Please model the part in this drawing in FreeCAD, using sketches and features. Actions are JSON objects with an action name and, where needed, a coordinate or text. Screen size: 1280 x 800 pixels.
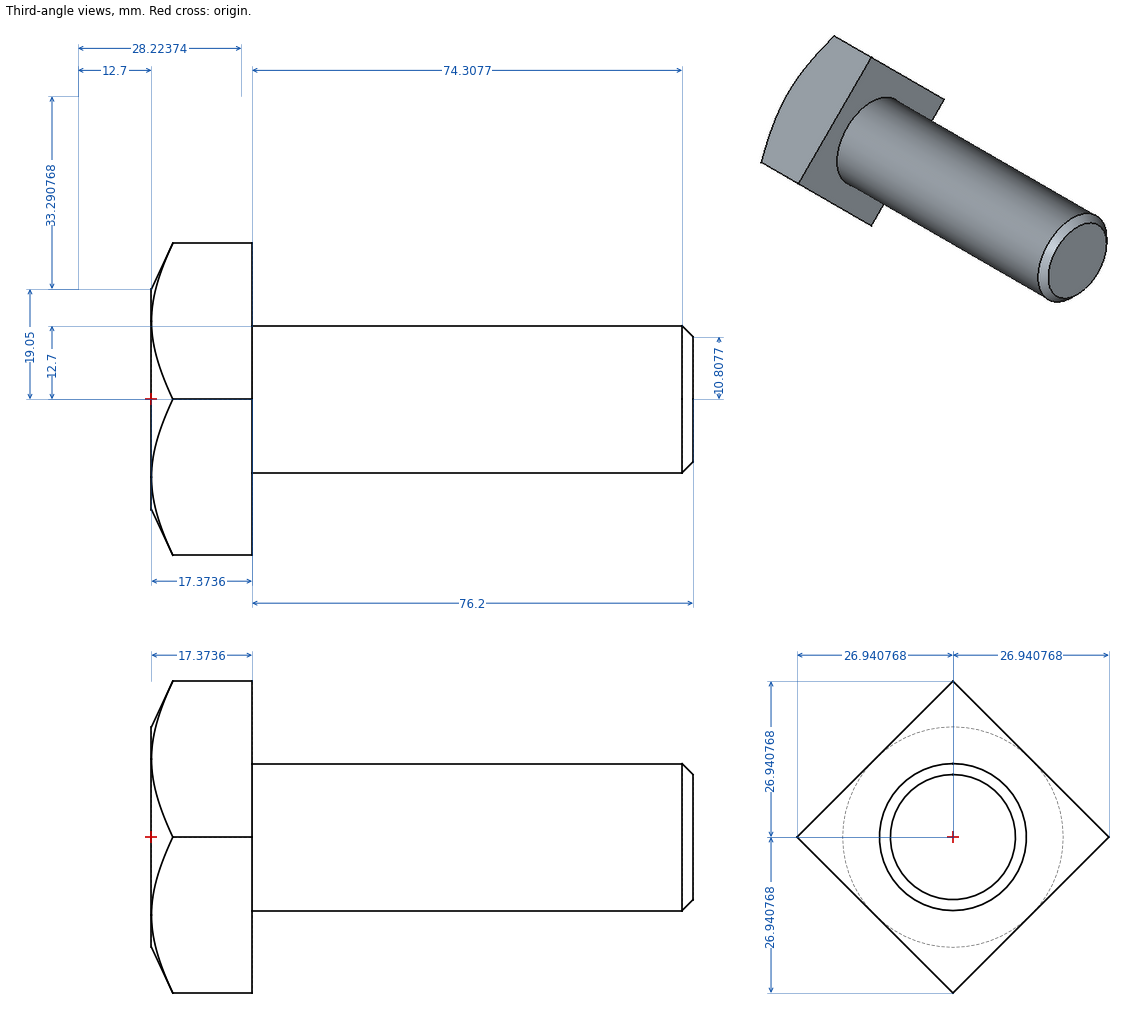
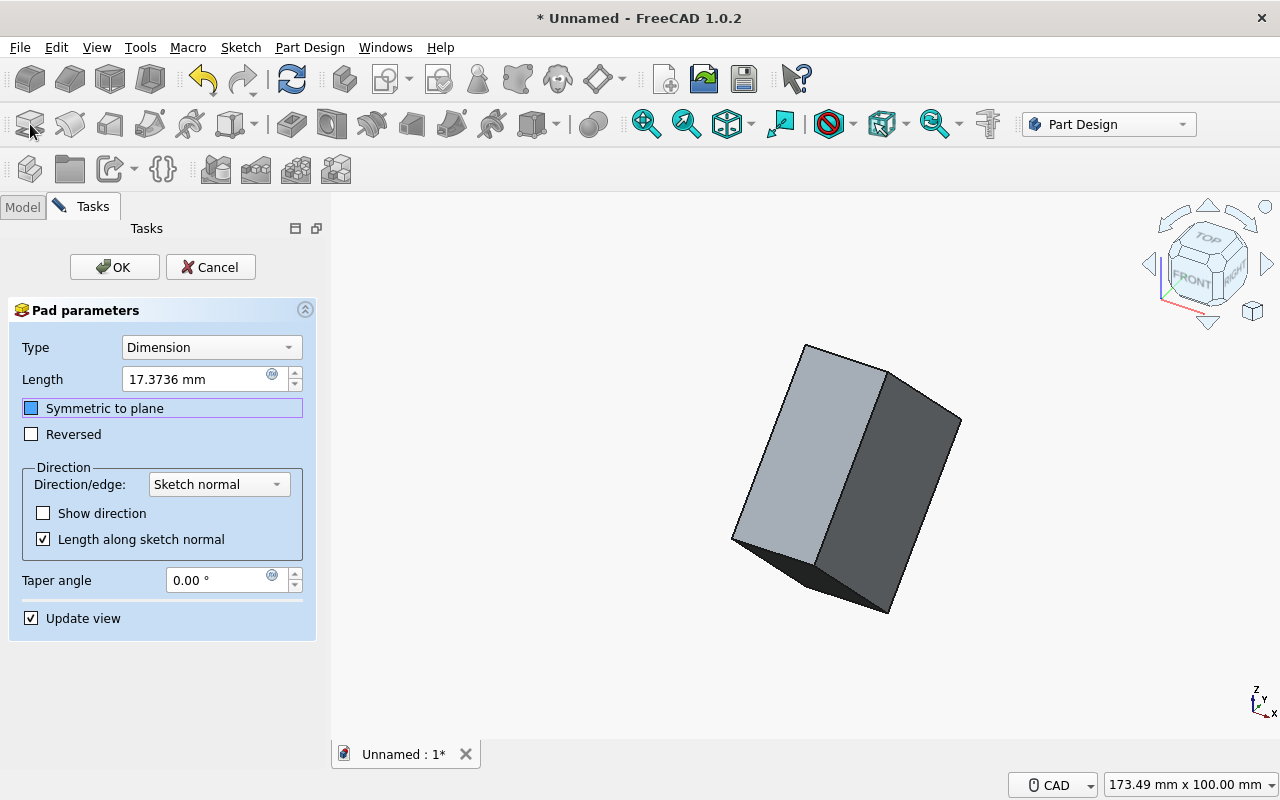
{"action": "left_click", "coordinate": [115, 267]}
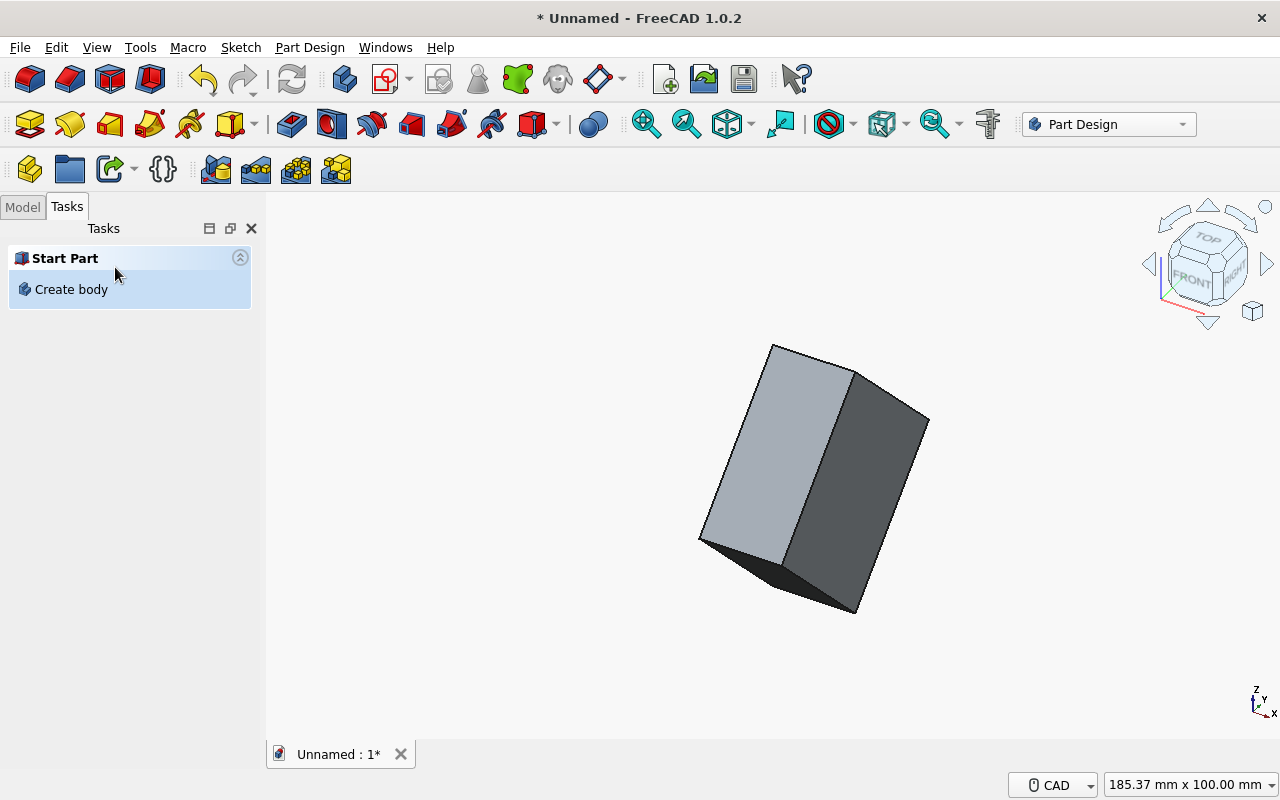
{"action": "left_click", "coordinate": [386, 80]}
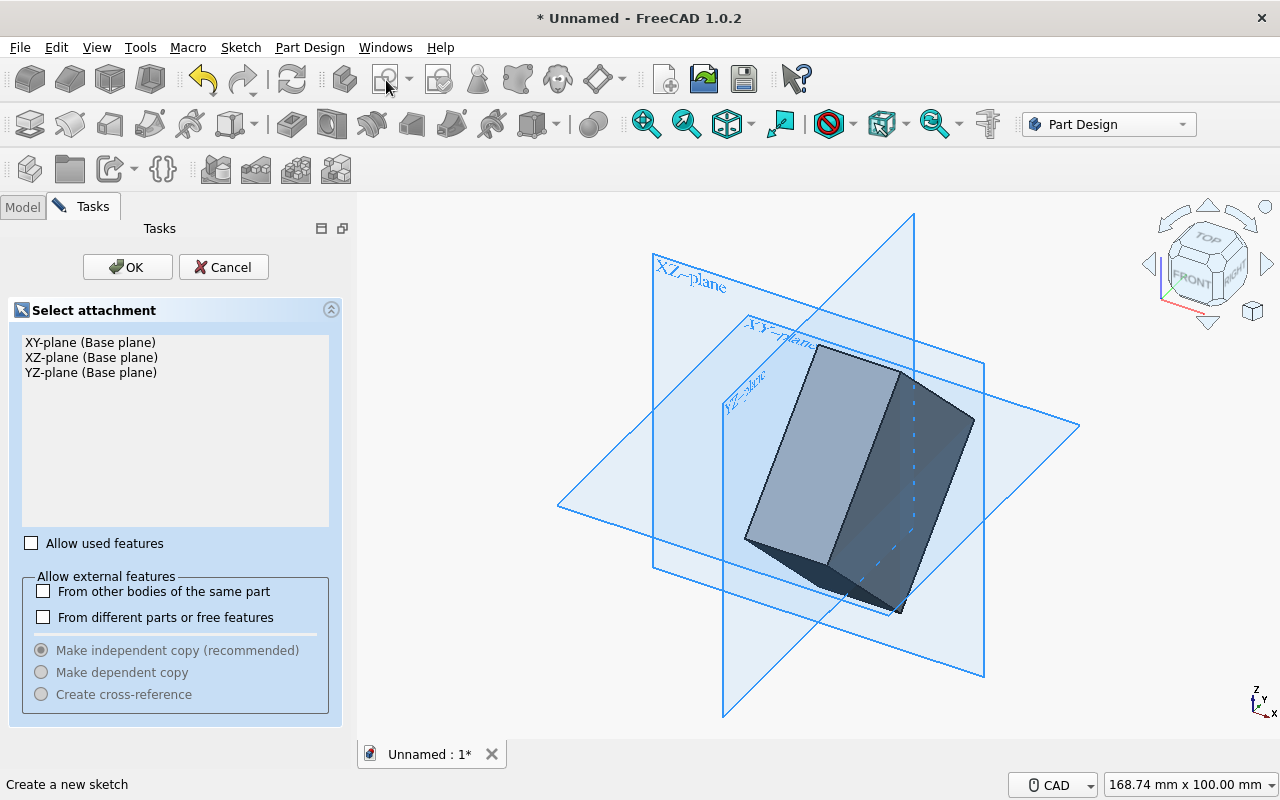
{"action": "left_click", "coordinate": [82, 342]}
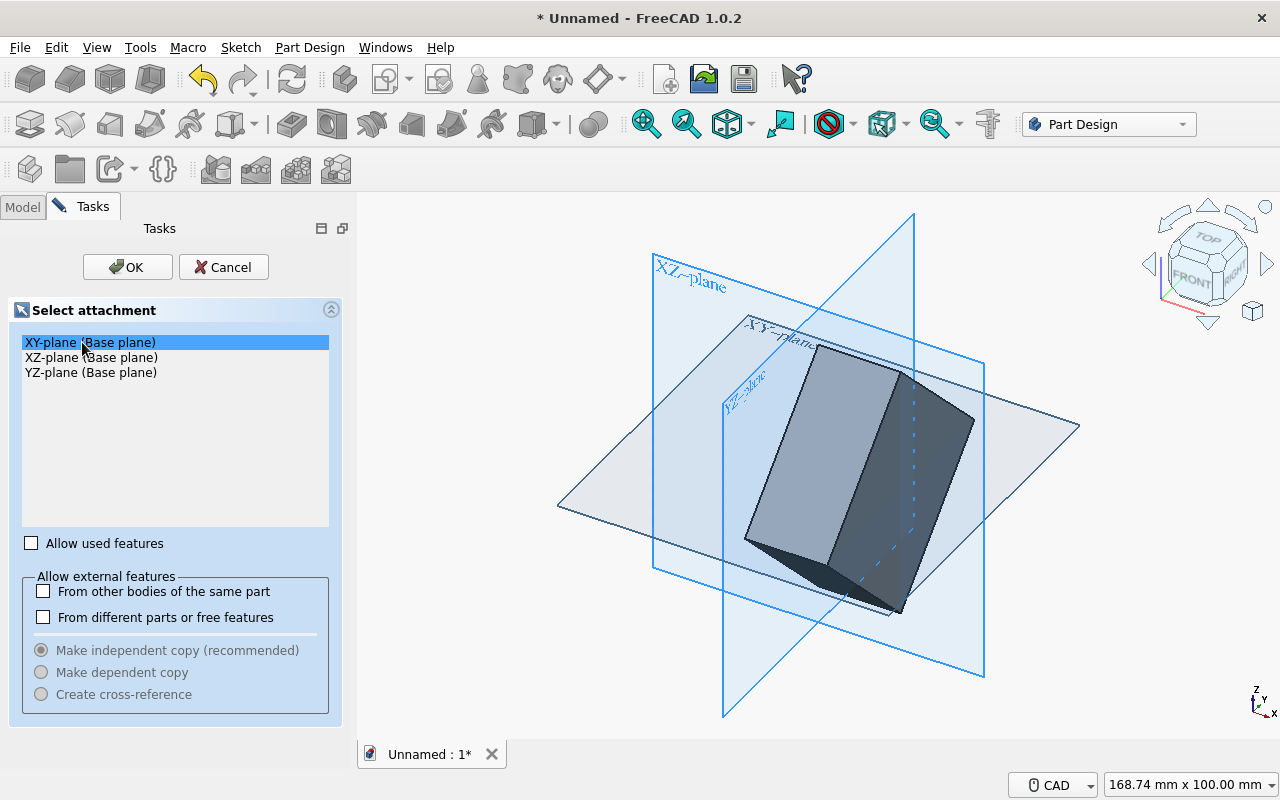
{"action": "left_click", "coordinate": [128, 267]}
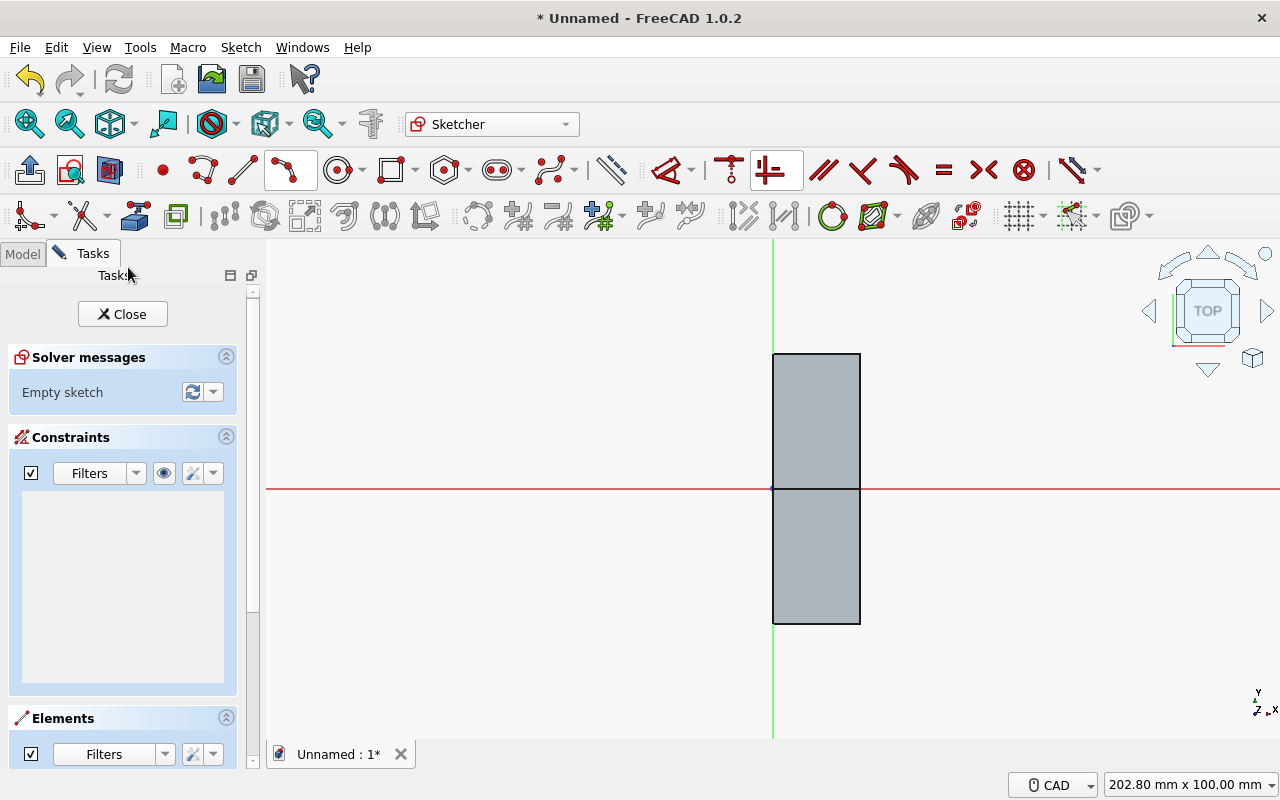
{"action": "key", "text": "q s"}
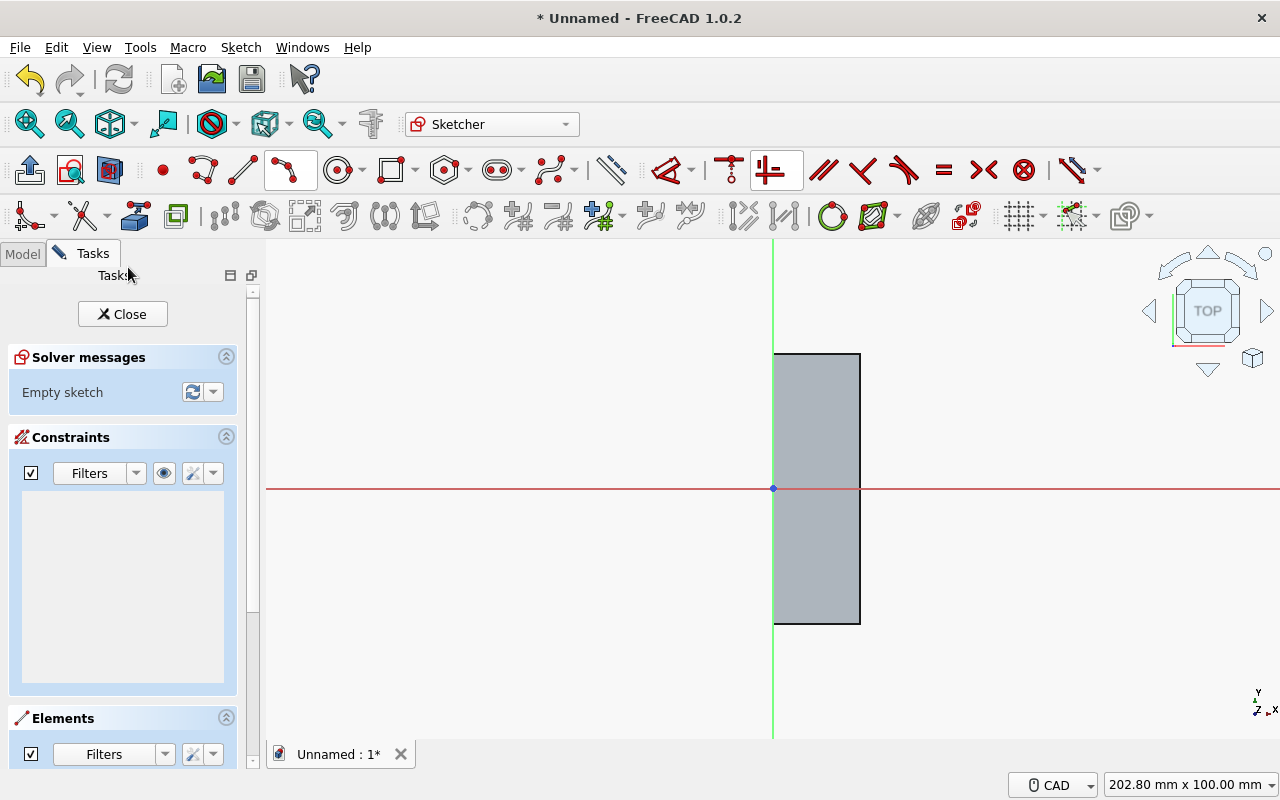
{"action": "scroll", "coordinate": [294, 632], "scroll_direction": "down", "scroll_amount": 1}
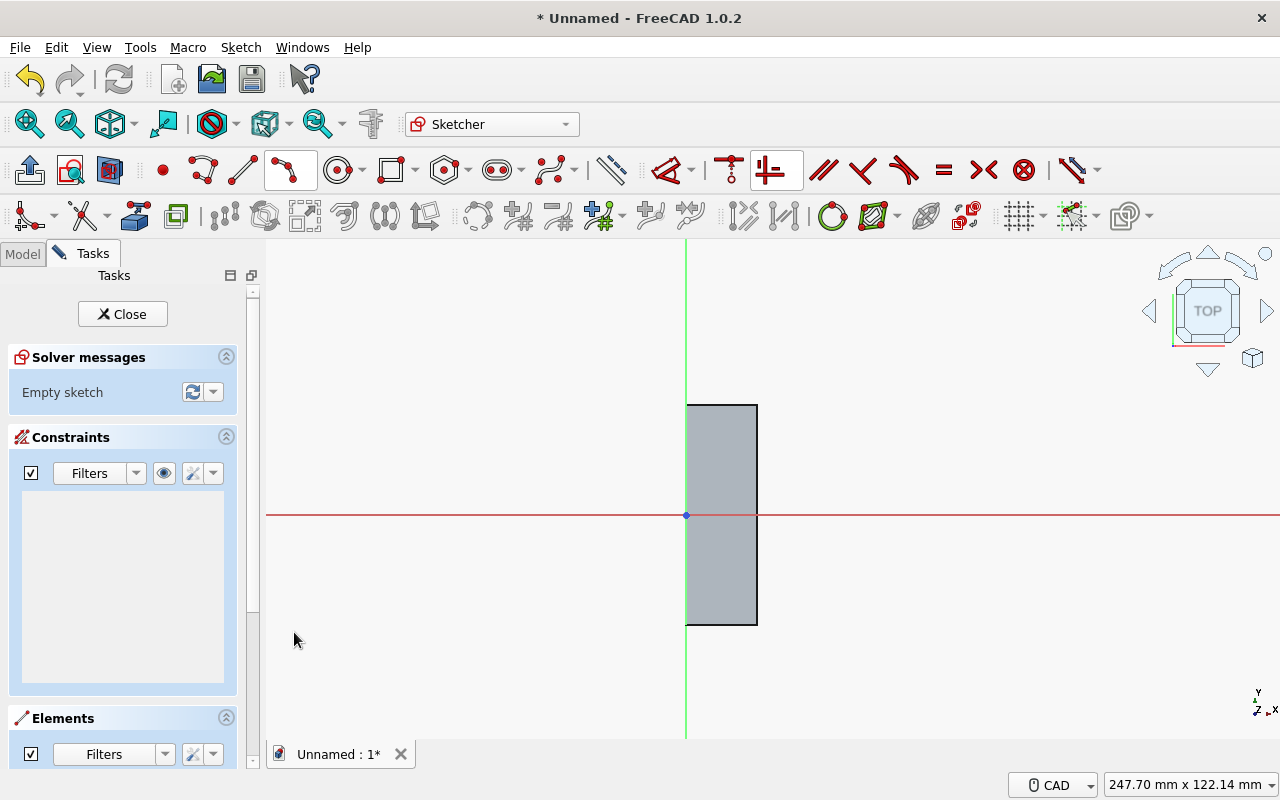
{"action": "scroll", "coordinate": [1115, 489], "scroll_direction": "up", "scroll_amount": 2}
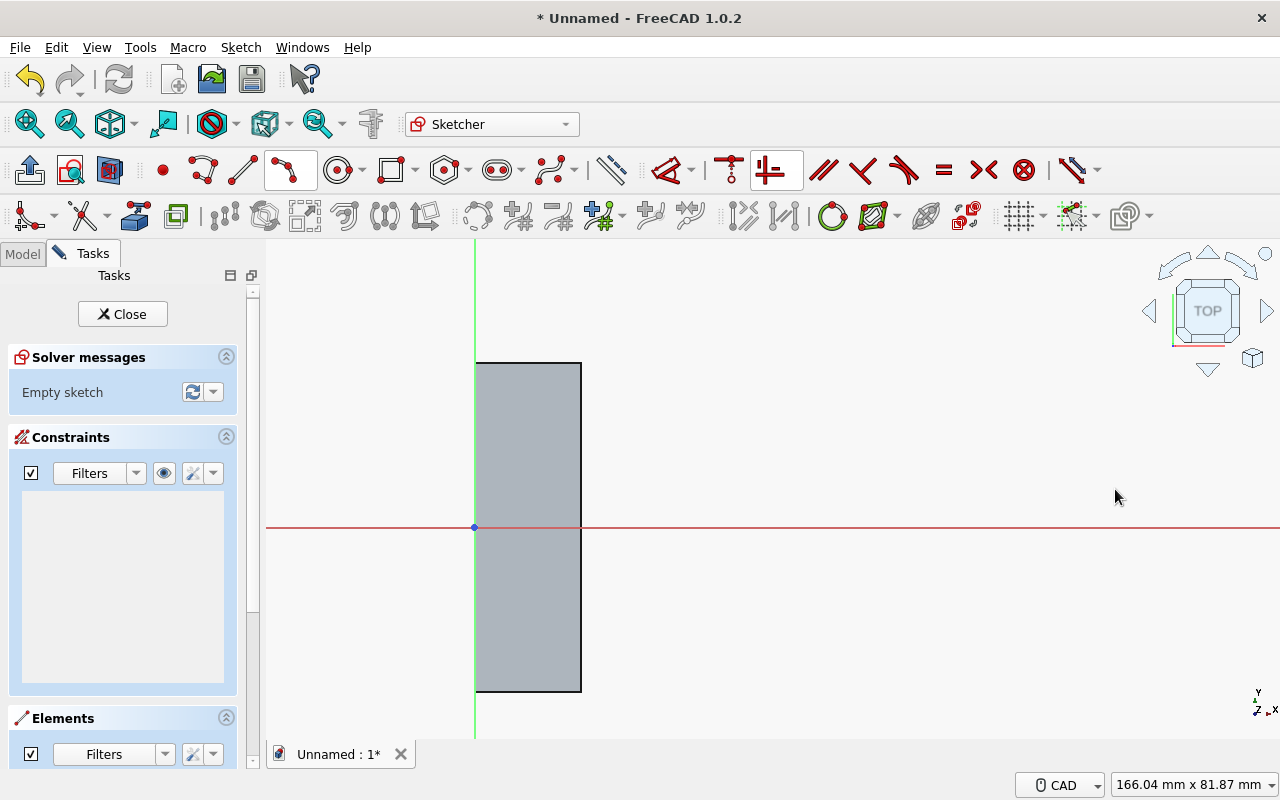
{"action": "left_click", "coordinate": [204, 170]}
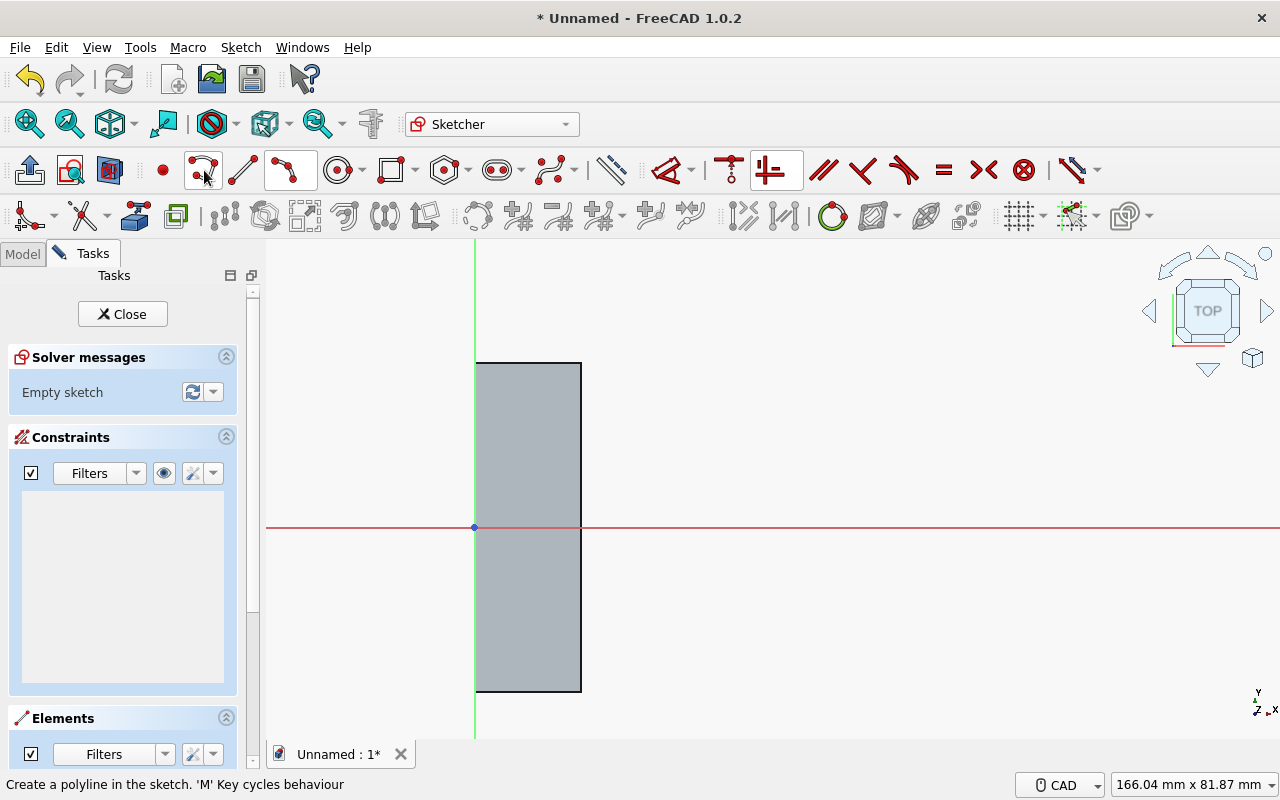
{"action": "left_click", "coordinate": [581, 528]}
{"action": "left_click", "coordinate": [1046, 519]}
{"action": "left_click", "coordinate": [1046, 462]}
{"action": "left_click", "coordinate": [1035, 450]}
{"action": "left_click", "coordinate": [581, 450]}
{"action": "left_click", "coordinate": [581, 528]}
{"action": "key", "text": "Escape"}
{"action": "key", "text": "Escape"}